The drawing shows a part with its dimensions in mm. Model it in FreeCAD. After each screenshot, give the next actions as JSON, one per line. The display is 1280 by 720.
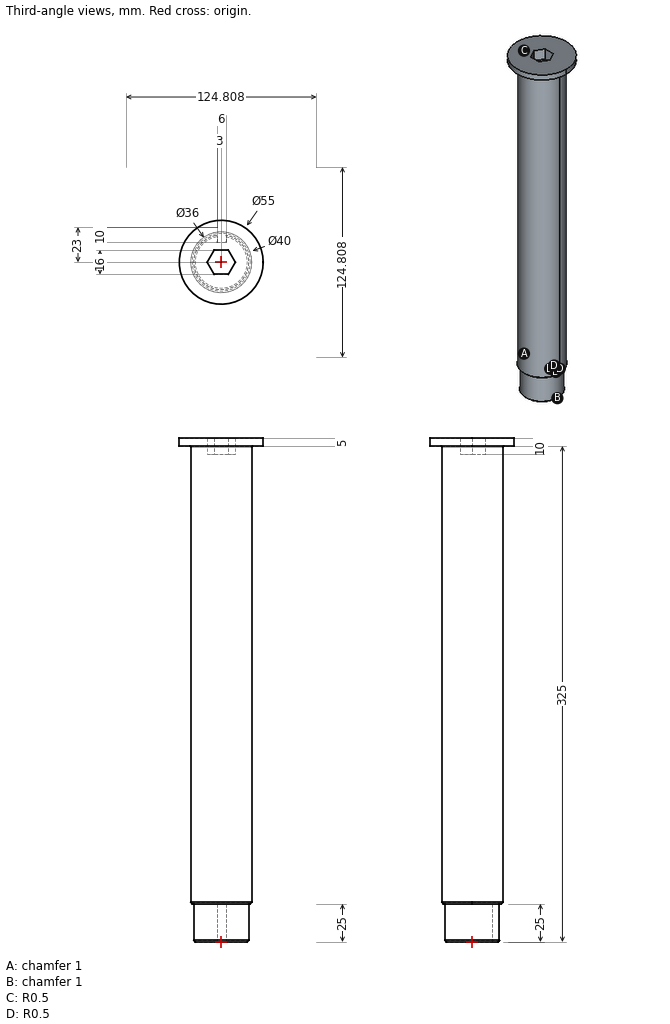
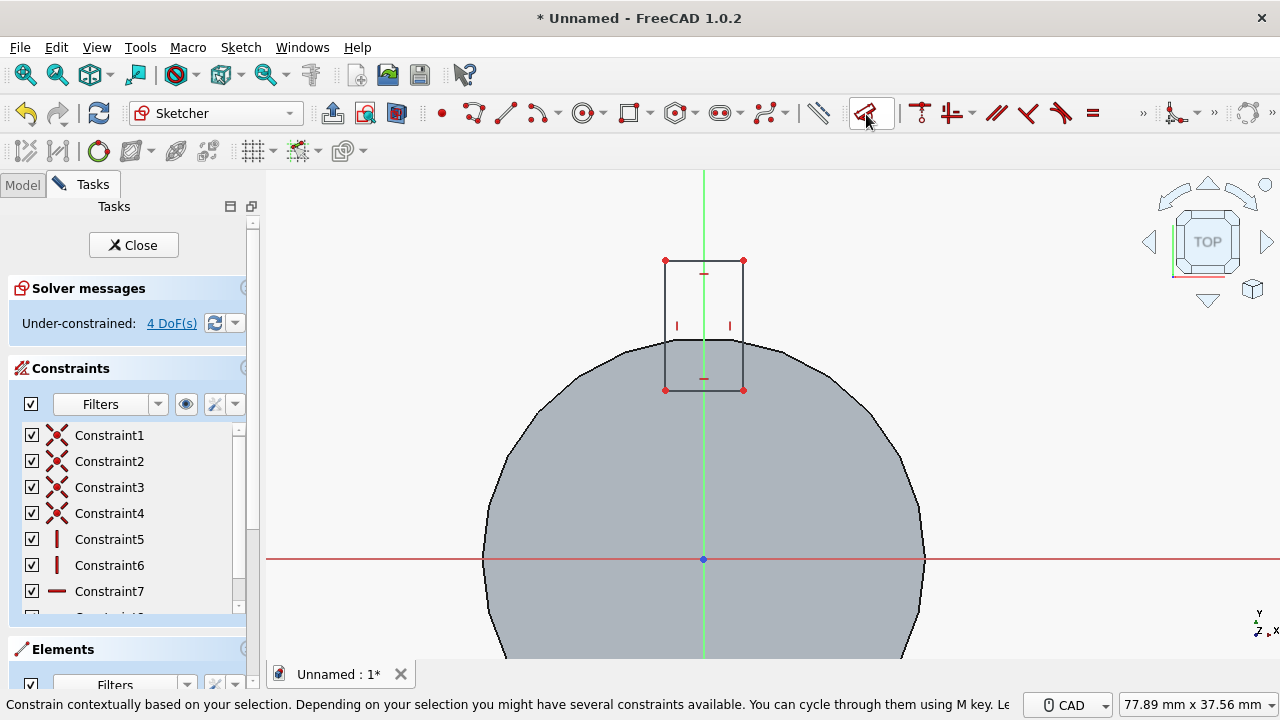
{"action": "left_click", "coordinate": [688, 391]}
{"action": "left_click", "coordinate": [686, 357]}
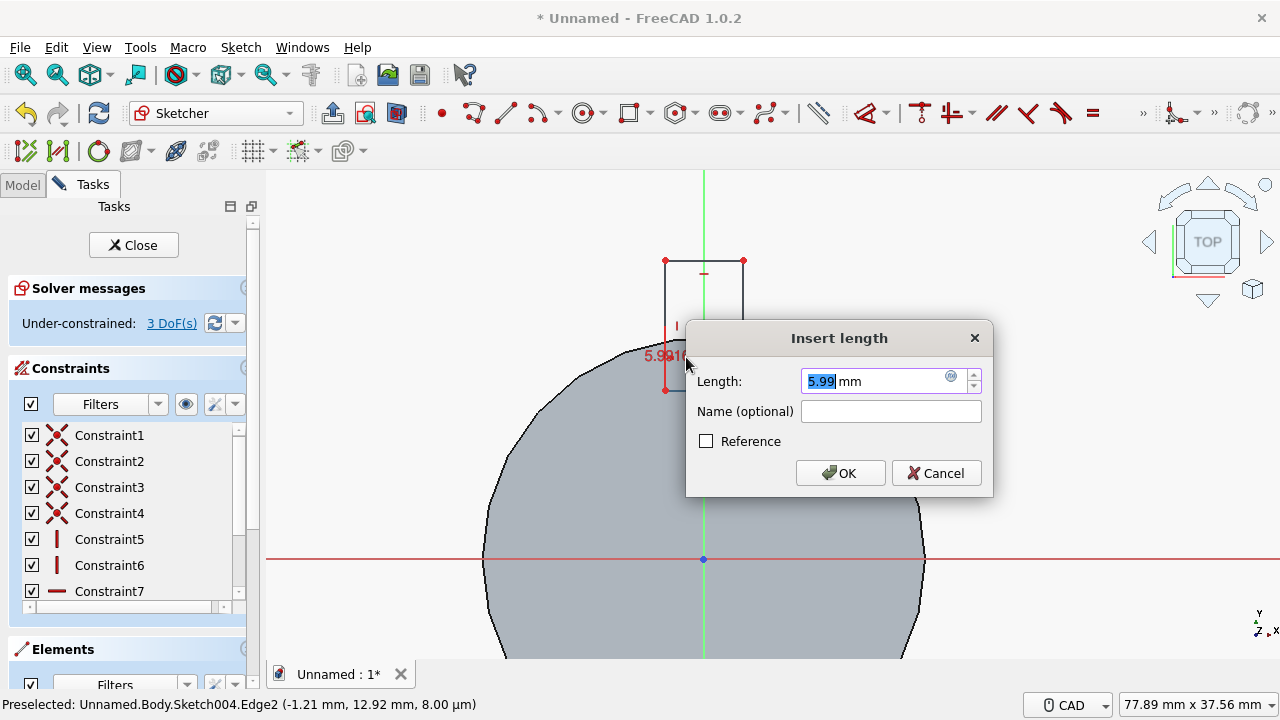
{"action": "type", "text": "6"}
{"action": "key", "text": "Return"}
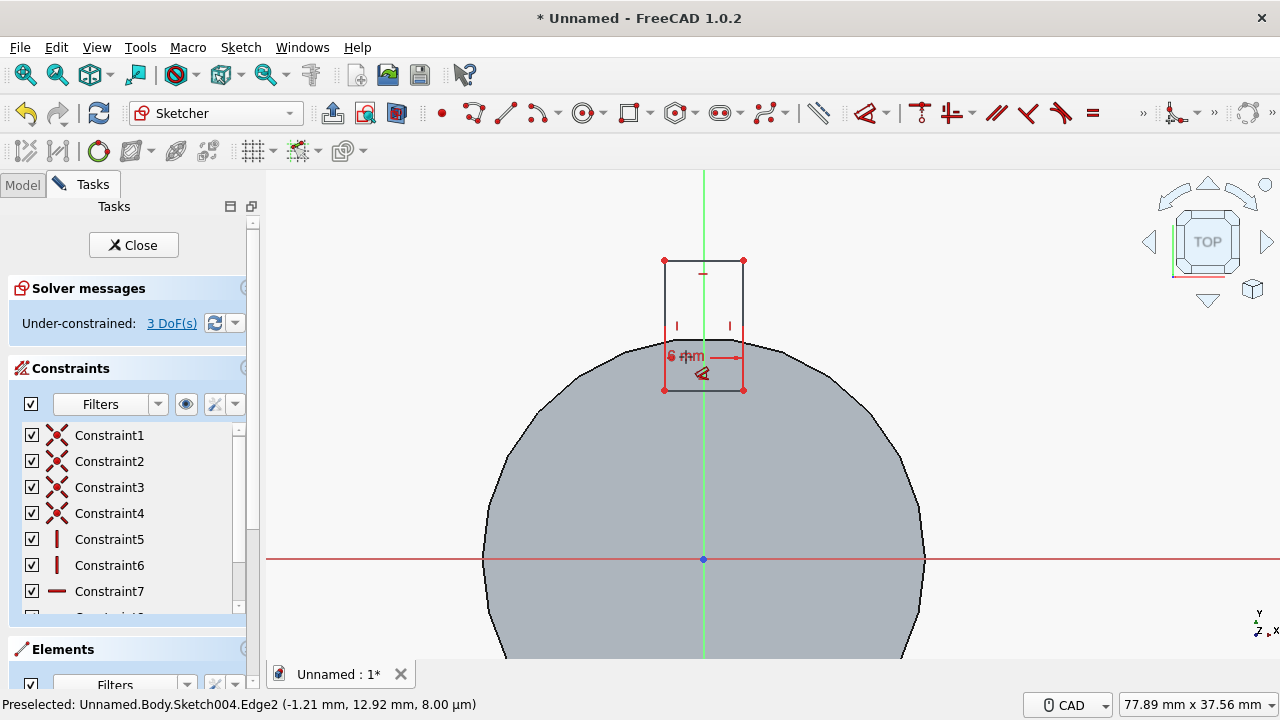
{"action": "left_click", "coordinate": [665, 300]}
{"action": "left_click", "coordinate": [631, 326]}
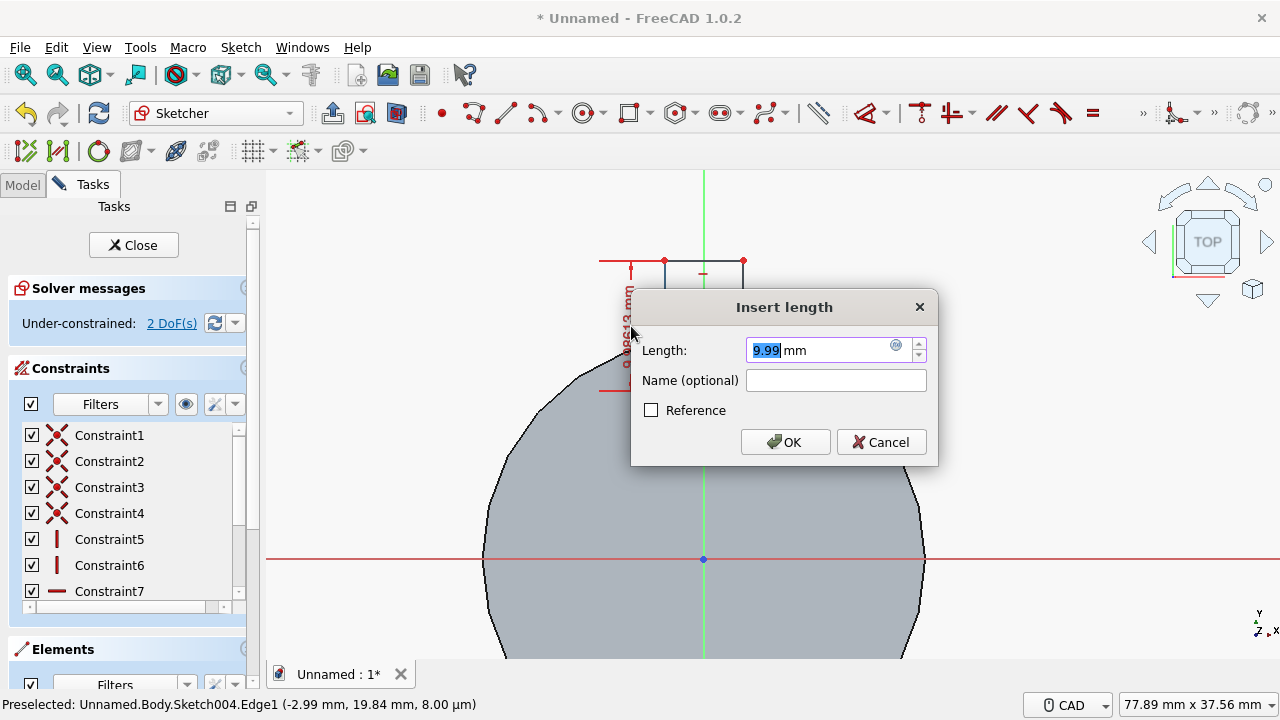
{"action": "type", "text": "10"}
{"action": "key", "text": "Return"}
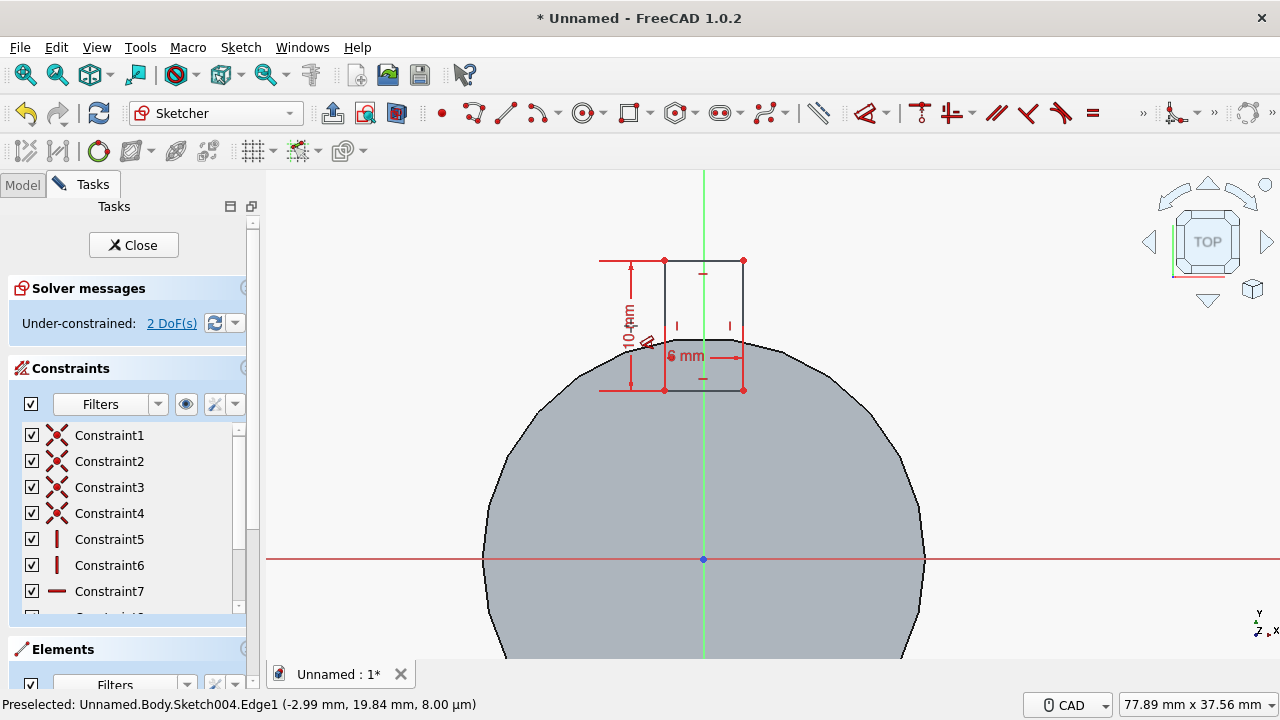
{"action": "left_click", "coordinate": [665, 261]}
{"action": "left_click", "coordinate": [684, 593]}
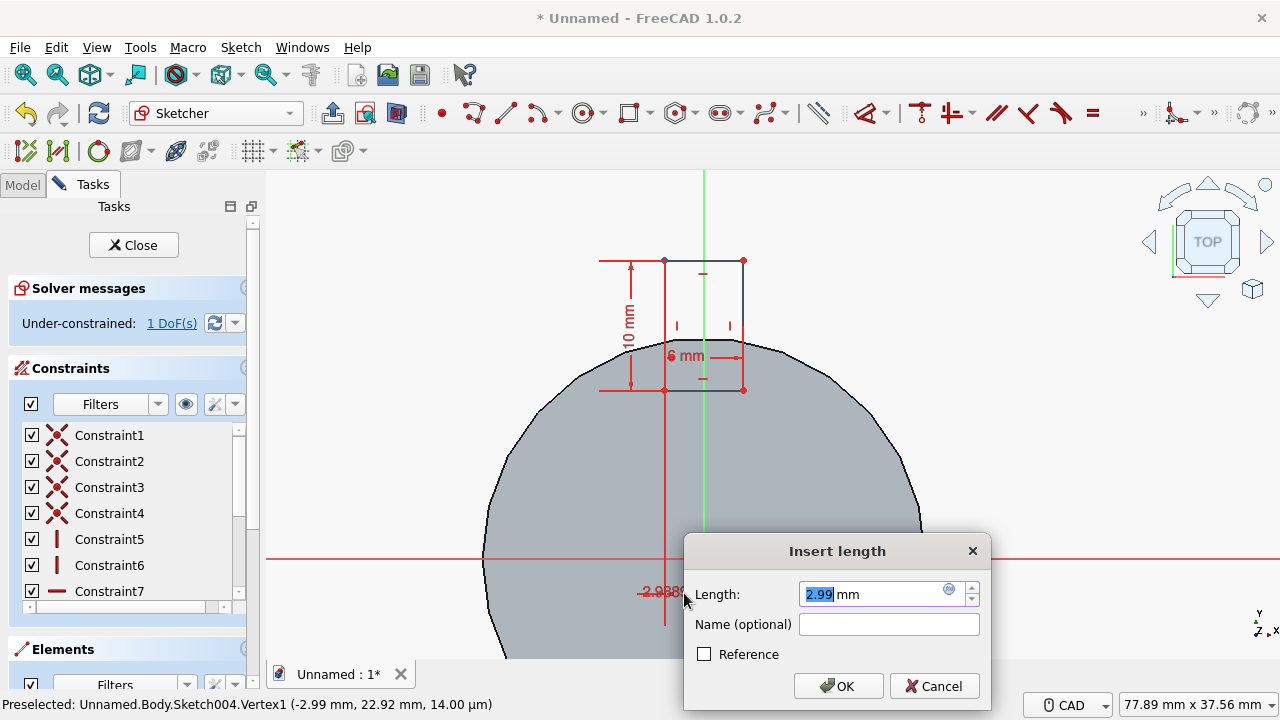
{"action": "type", "text": "3"}
{"action": "key", "text": "Return"}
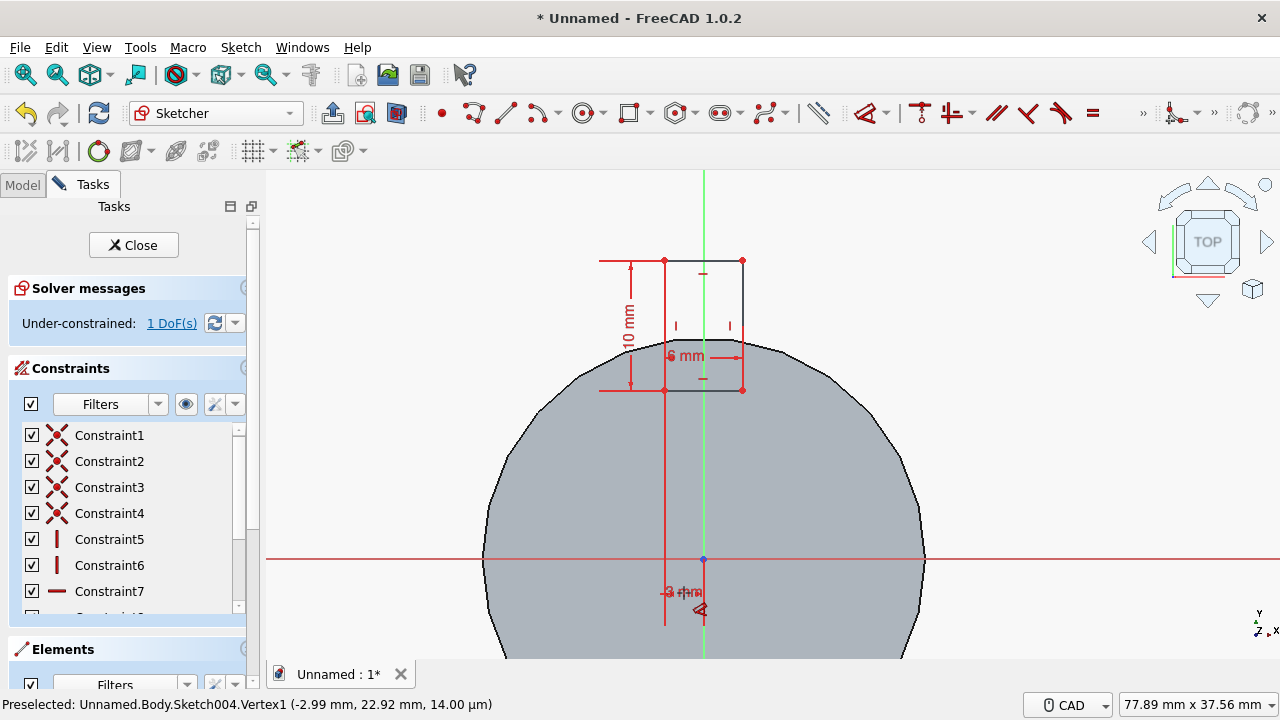
{"action": "left_click", "coordinate": [665, 261]}
{"action": "left_click", "coordinate": [631, 410]}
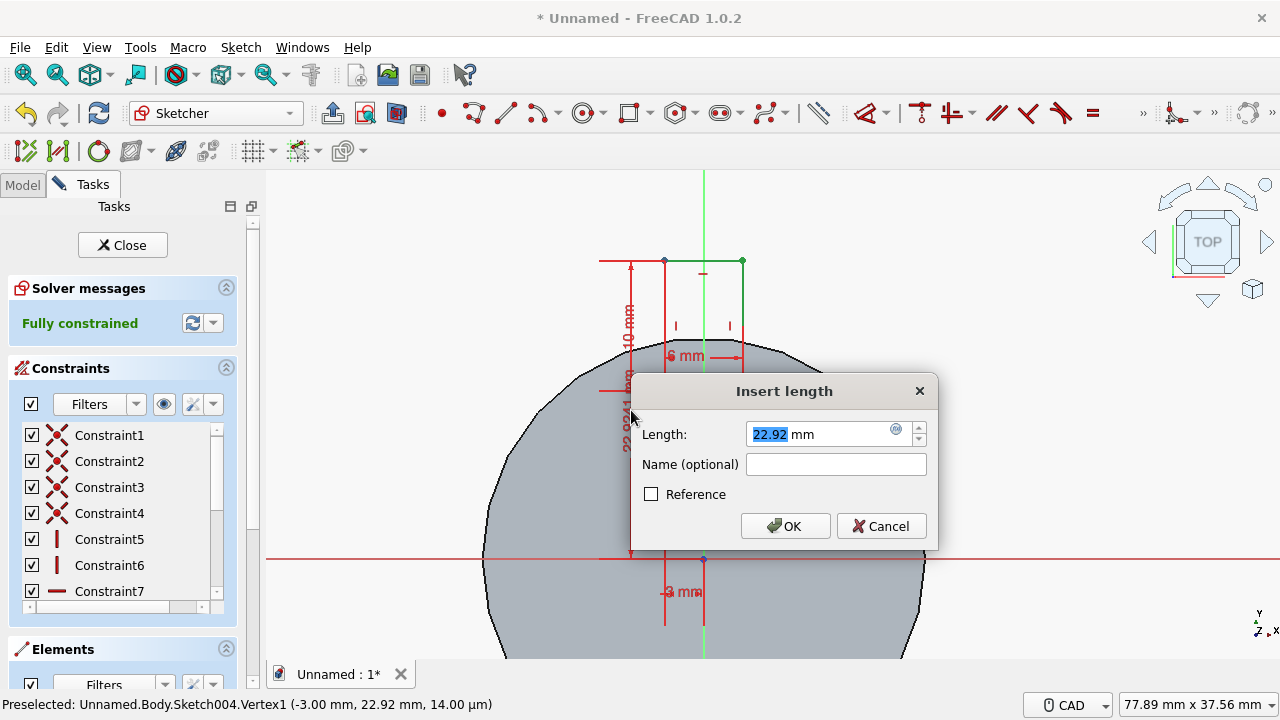
{"action": "type", "text": "23"}
{"action": "key", "text": "Return"}
{"action": "key", "text": "Escape"}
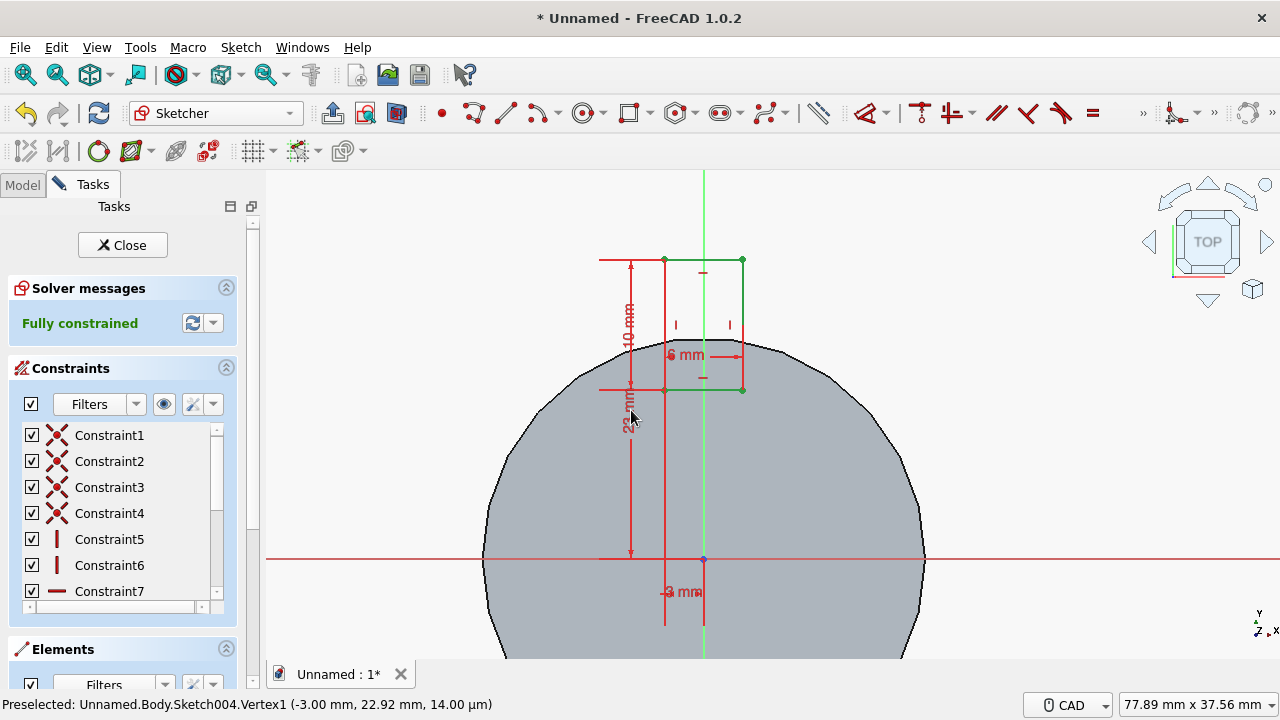
{"action": "left_click", "coordinate": [123, 245]}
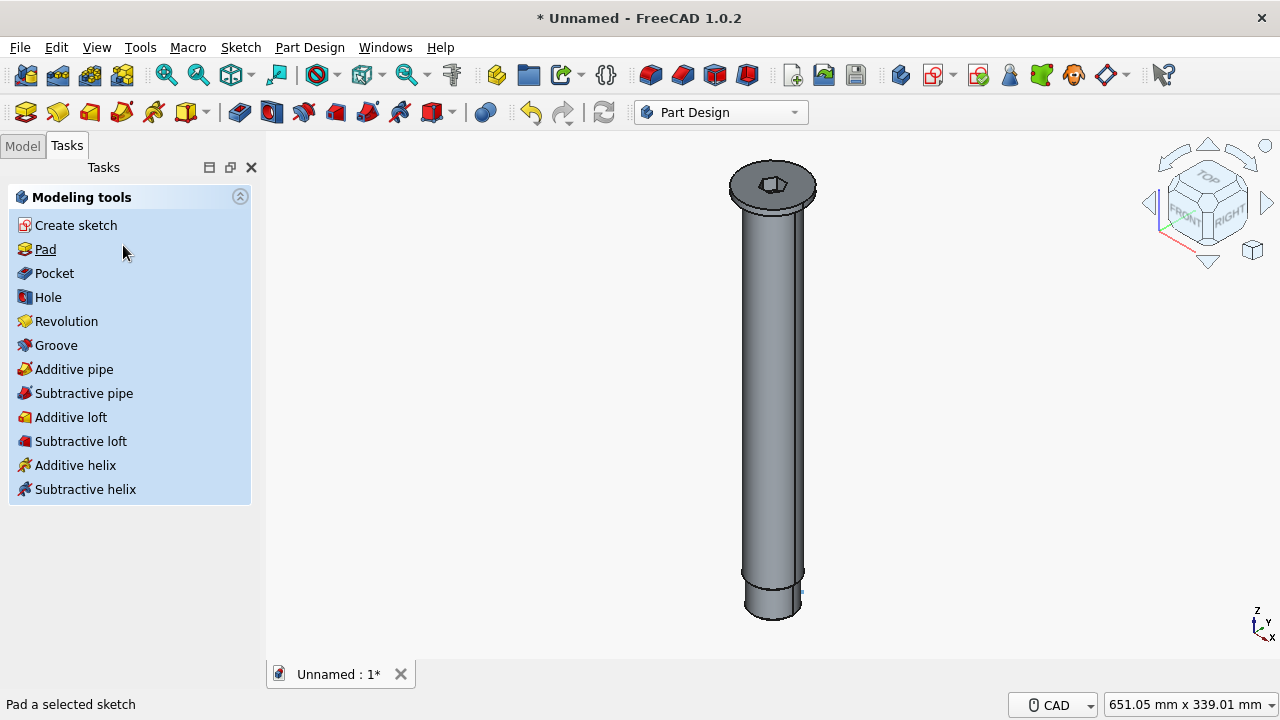
{"action": "left_click", "coordinate": [240, 112]}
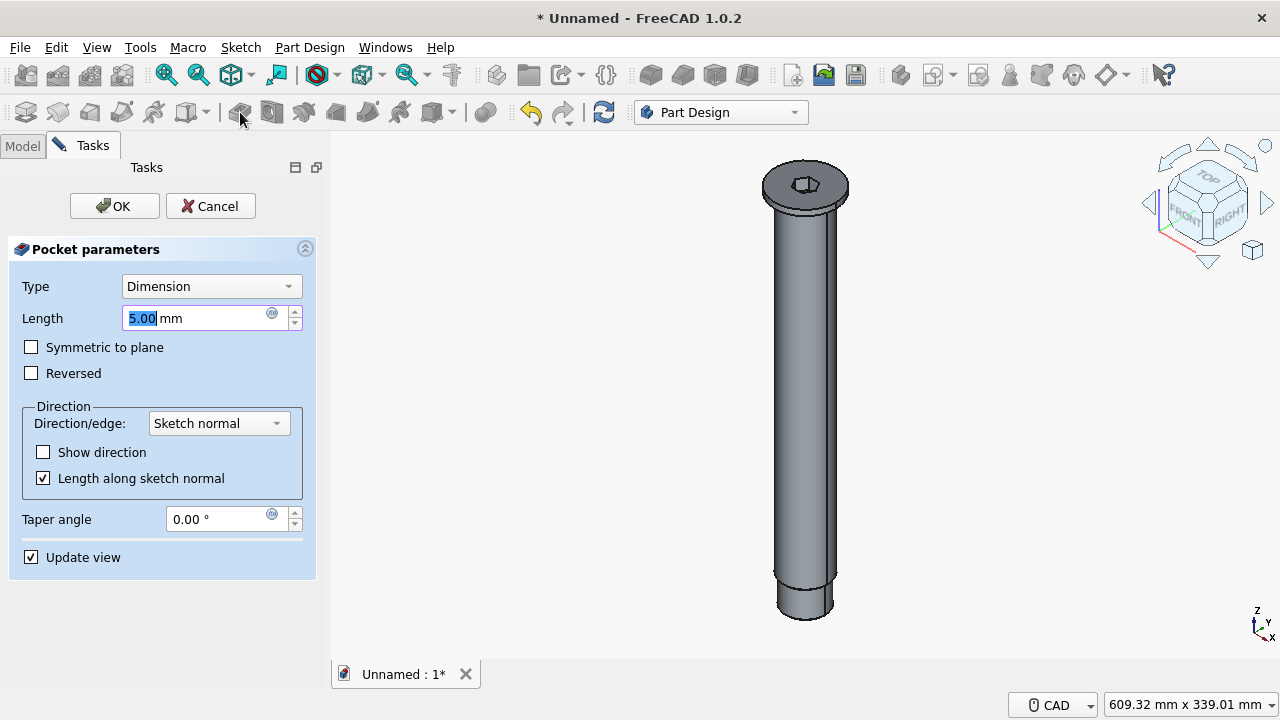
{"action": "type", "text": "25"}
{"action": "key", "text": "Tab"}